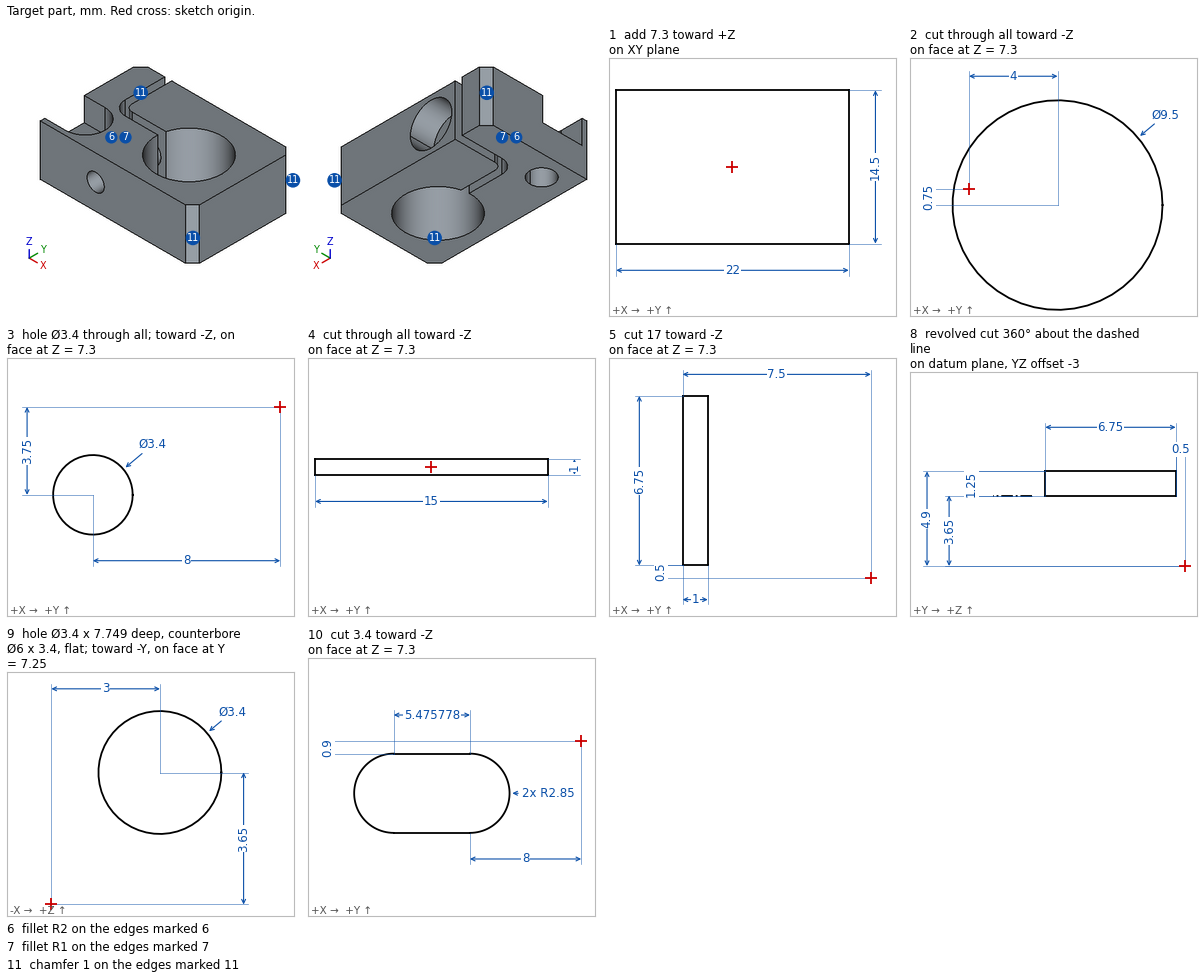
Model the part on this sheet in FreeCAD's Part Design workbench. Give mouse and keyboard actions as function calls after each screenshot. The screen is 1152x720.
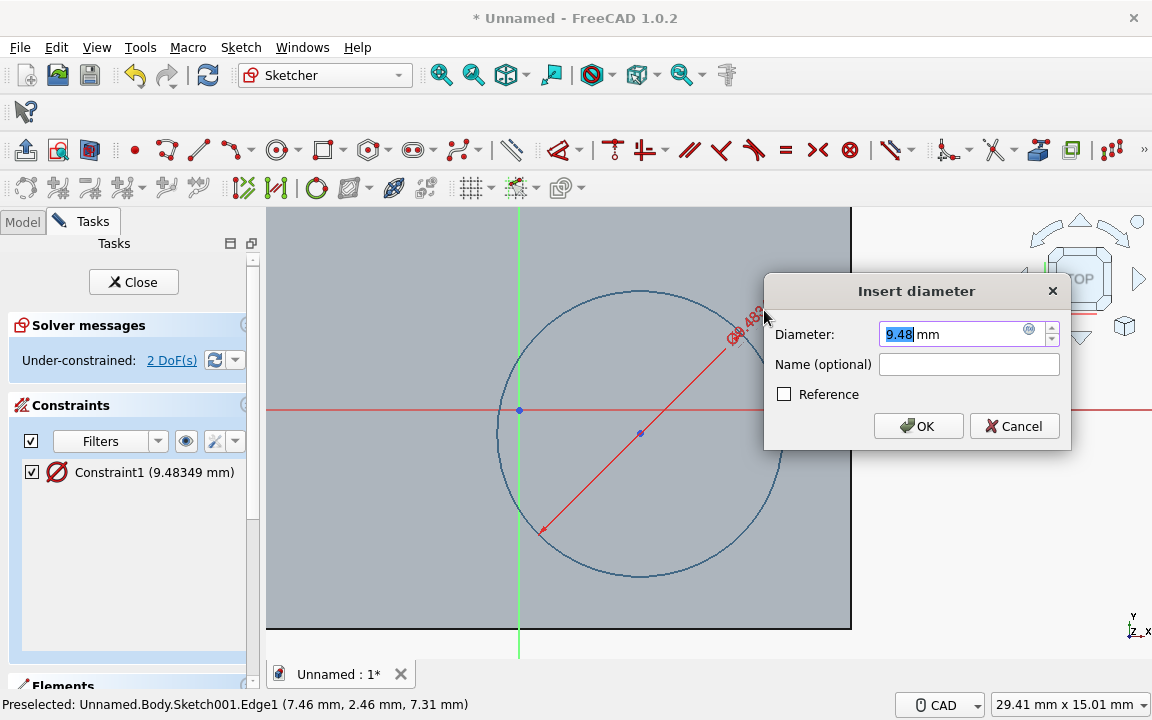
text(9.5)
key(Return)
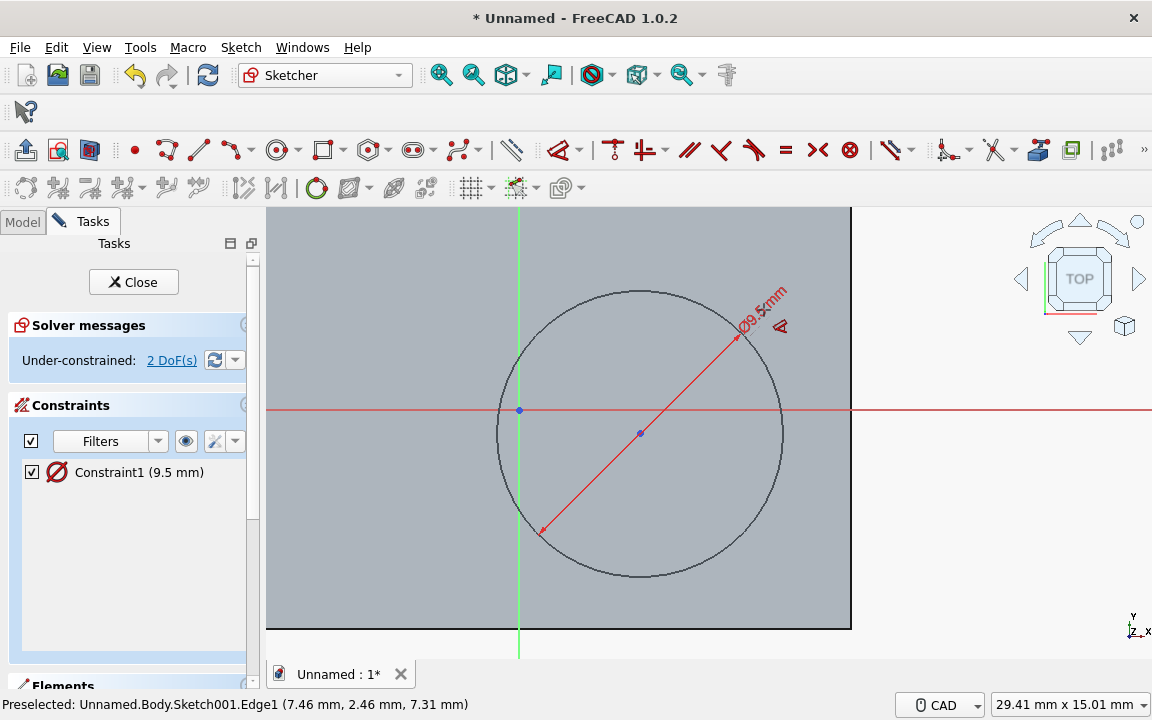
click(640, 434)
click(580, 376)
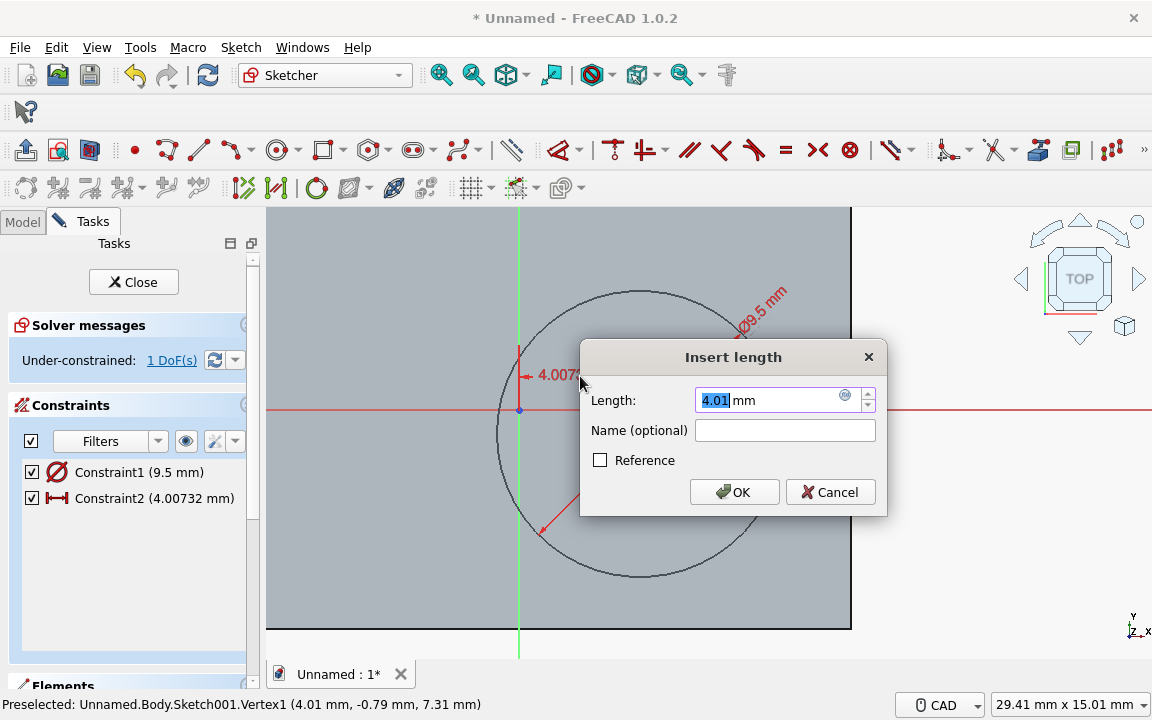
text(4)
key(Return)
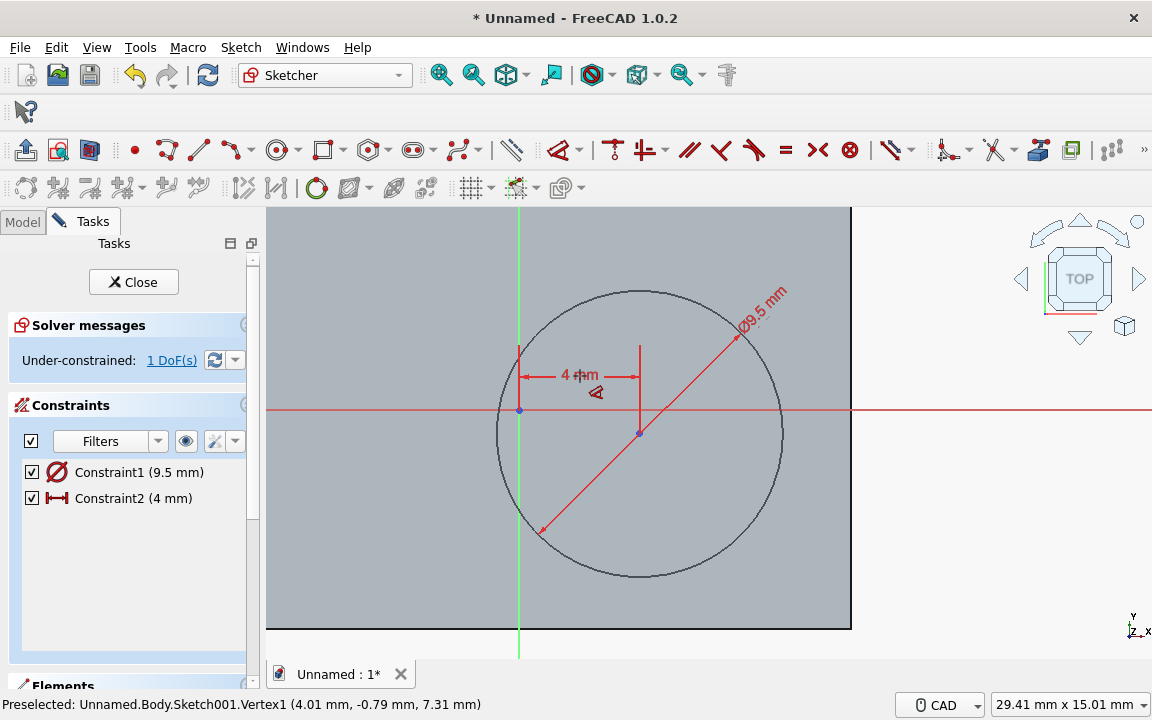
scroll(640, 434, up, 3)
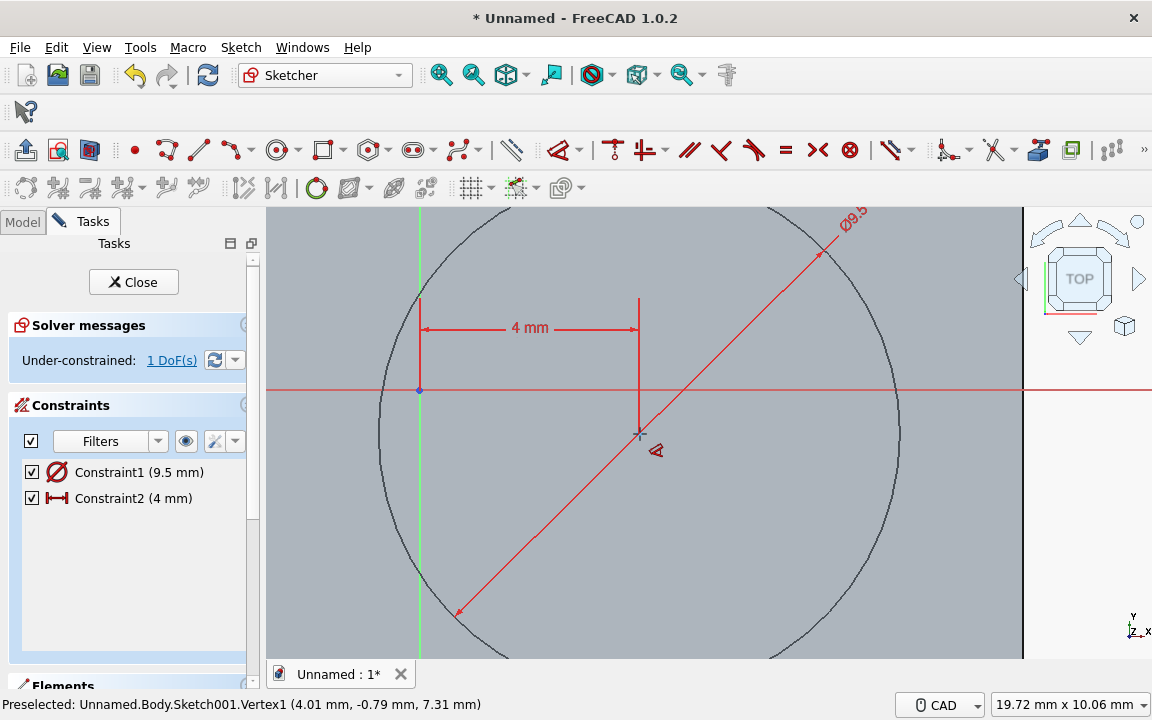
click(639, 434)
click(673, 412)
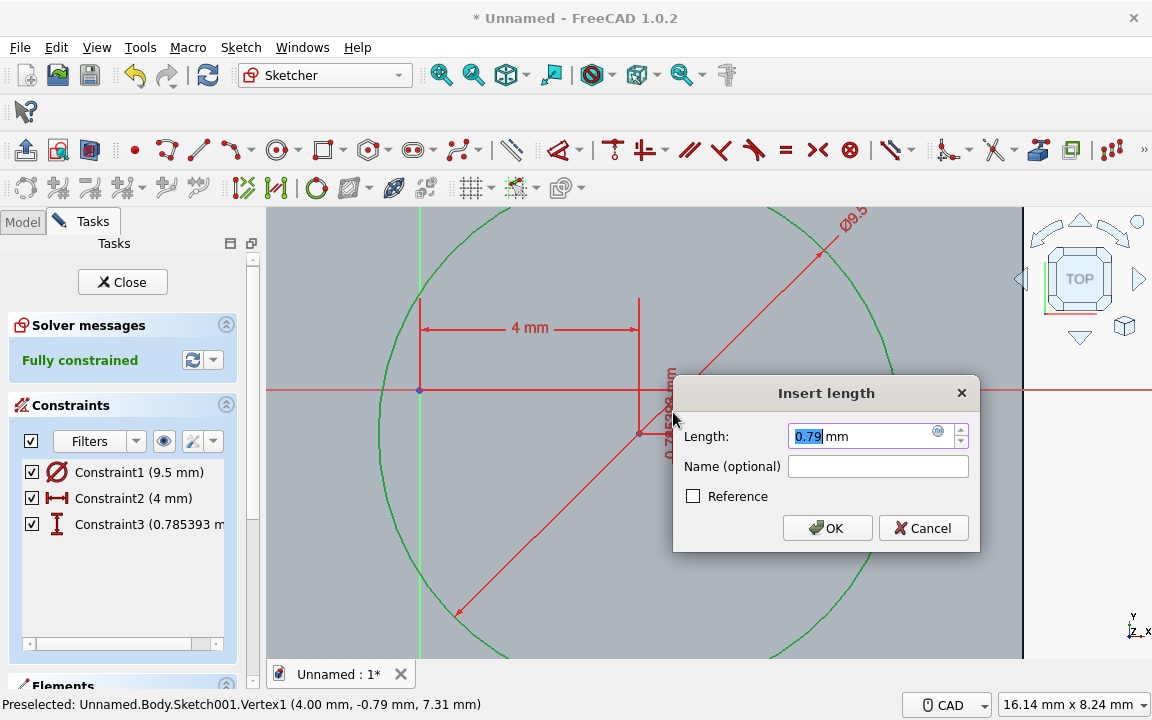
text(0.75)
key(Return)
key(Escape)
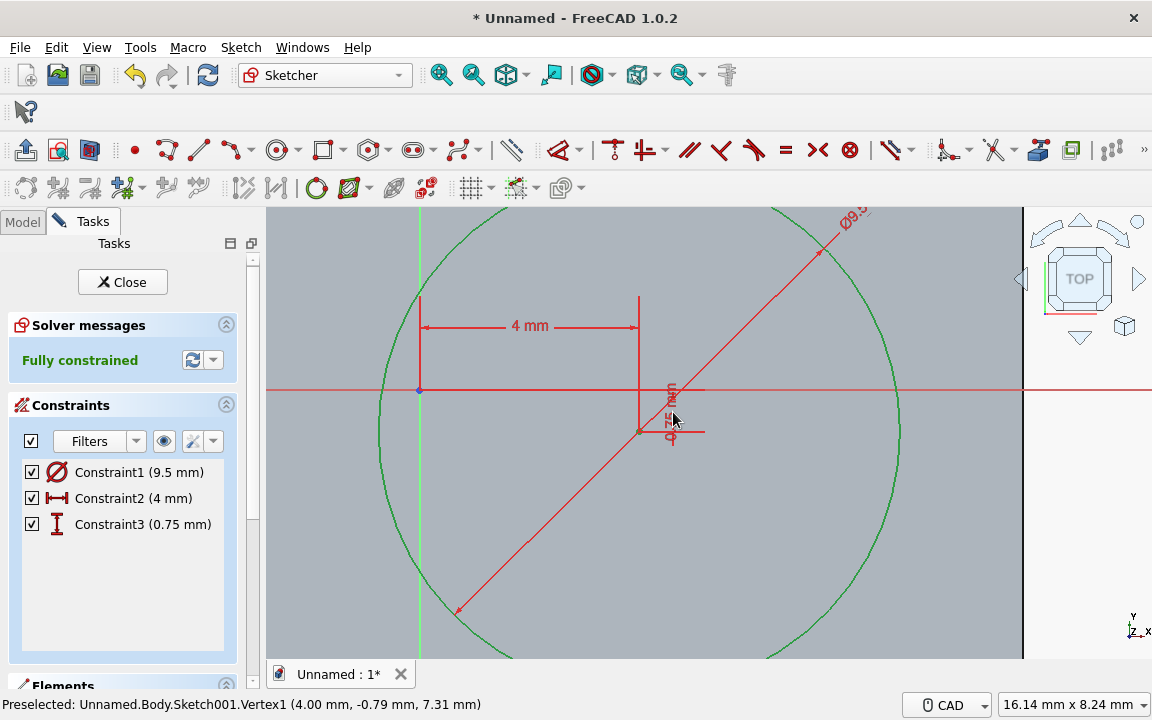
click(123, 282)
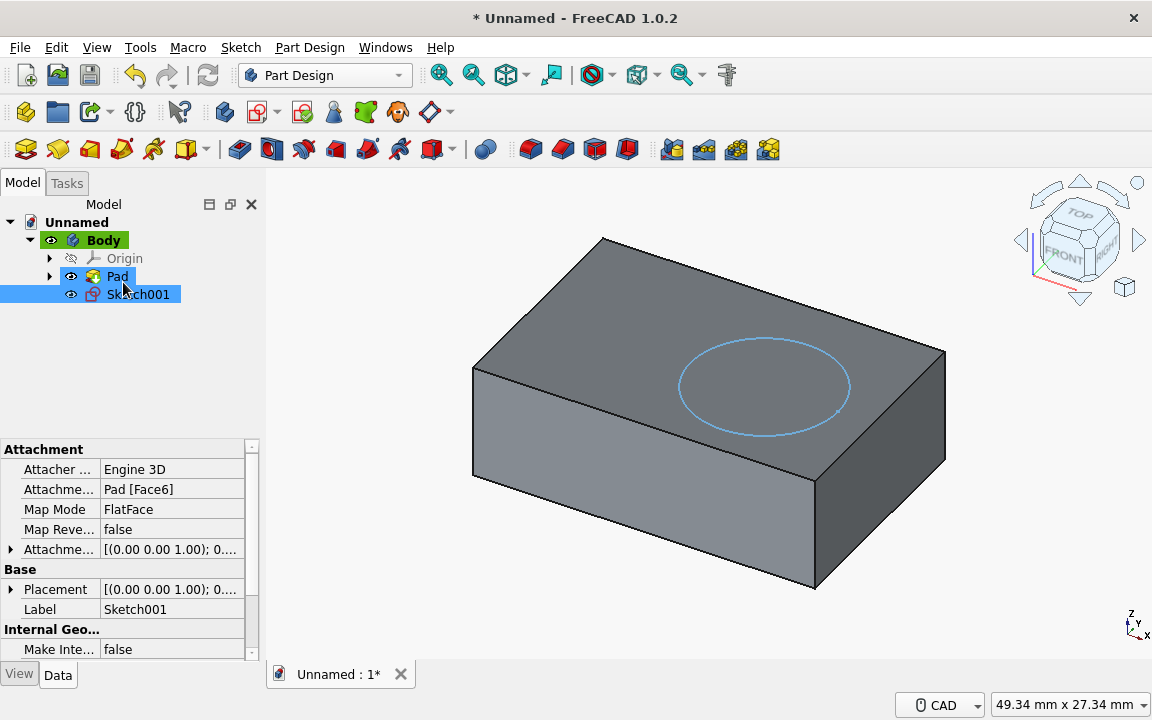
click(240, 150)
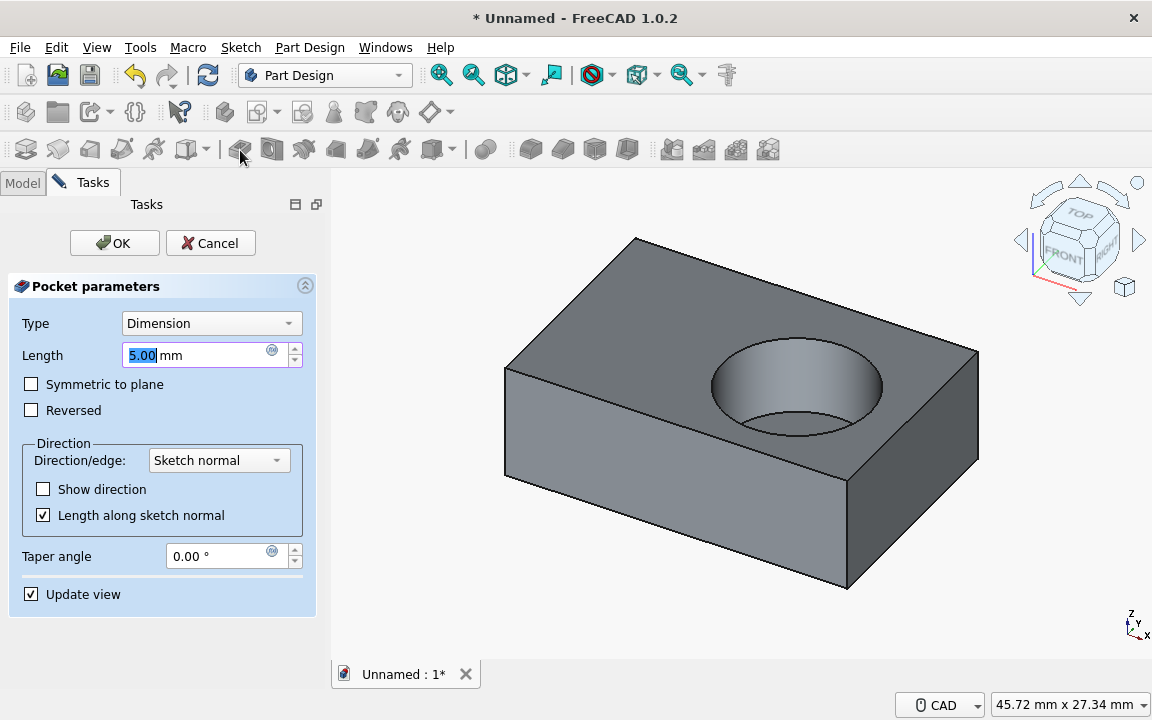
click(212, 324)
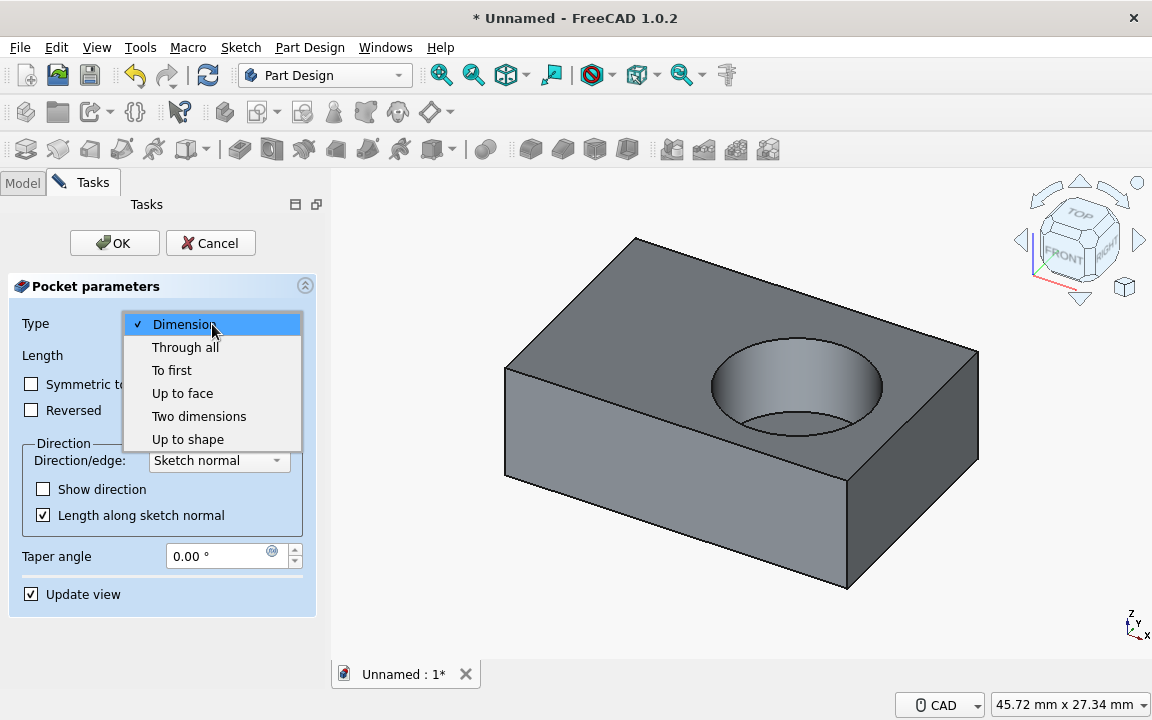
click(212, 348)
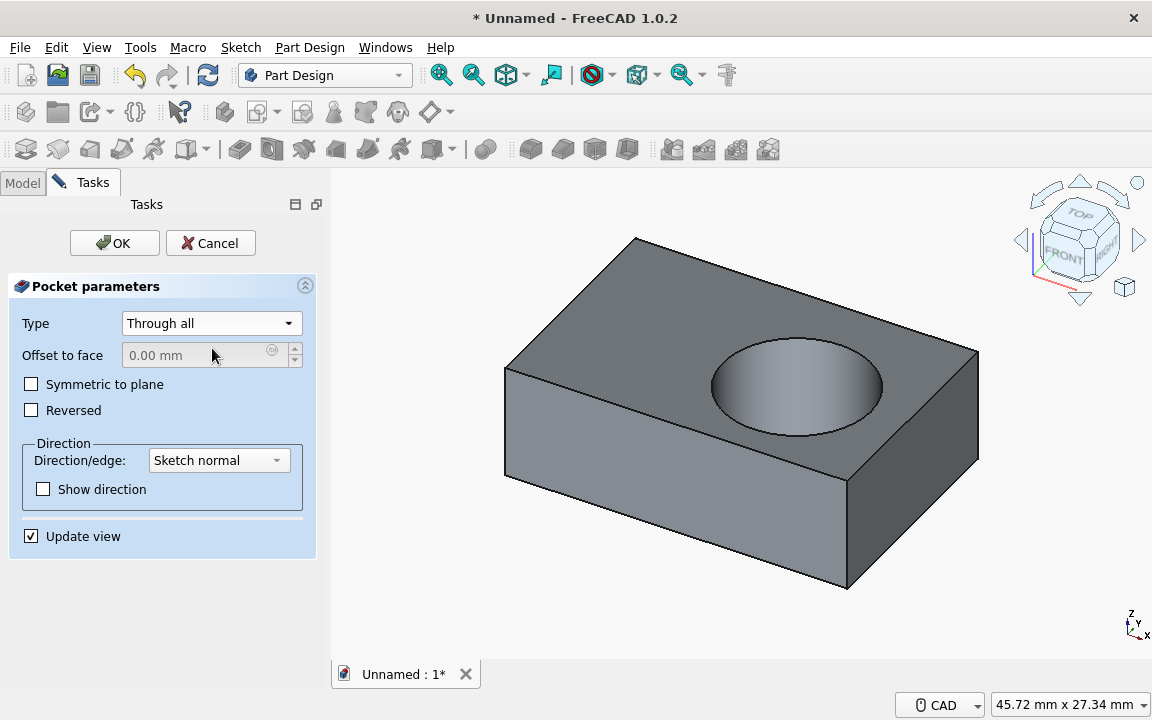
click(115, 243)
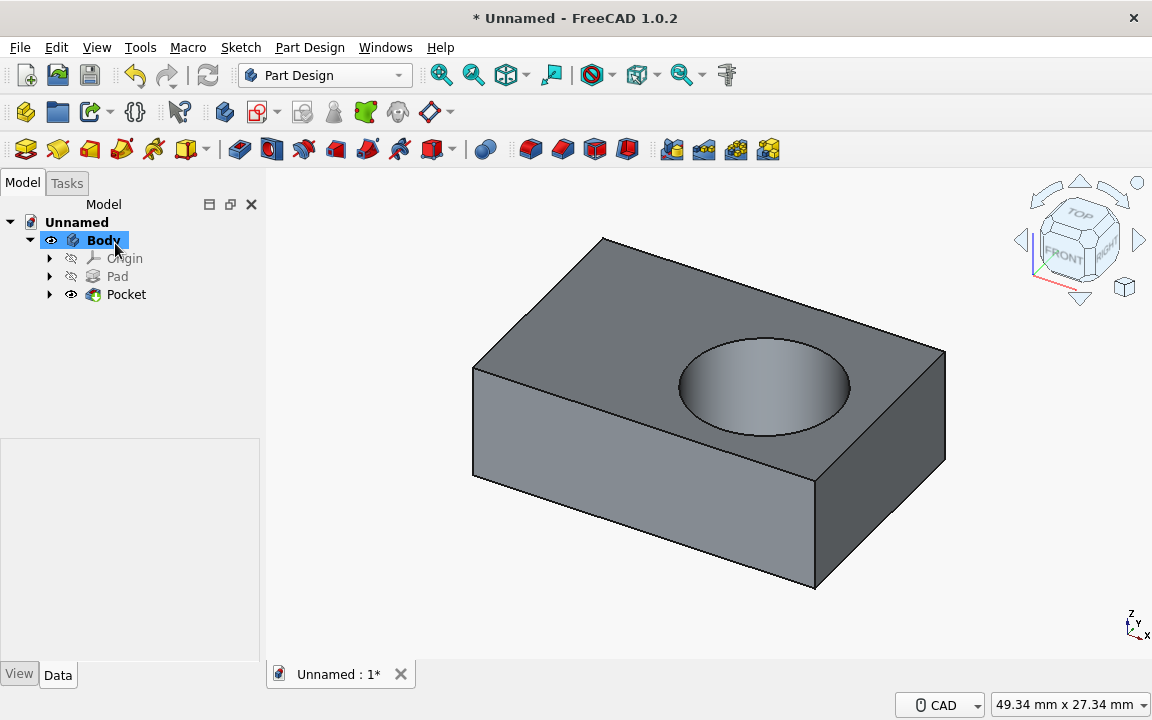
click(630, 308)